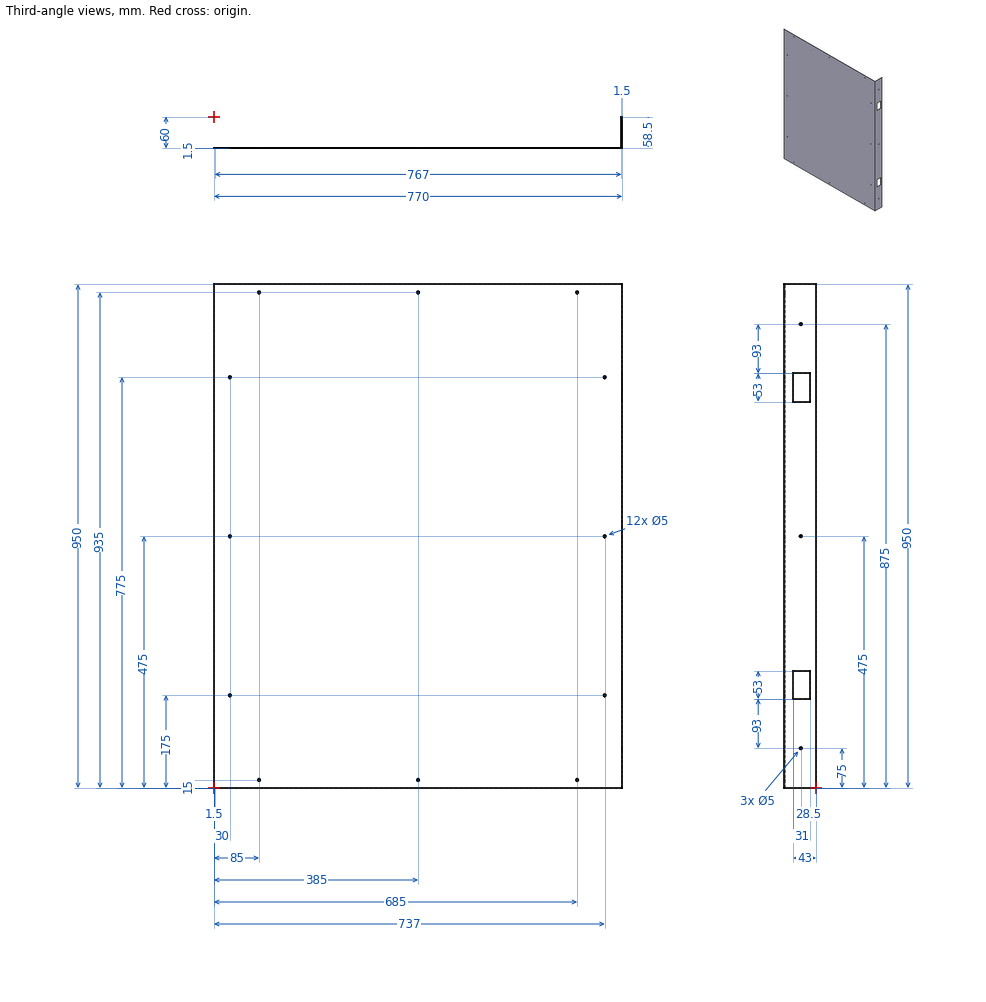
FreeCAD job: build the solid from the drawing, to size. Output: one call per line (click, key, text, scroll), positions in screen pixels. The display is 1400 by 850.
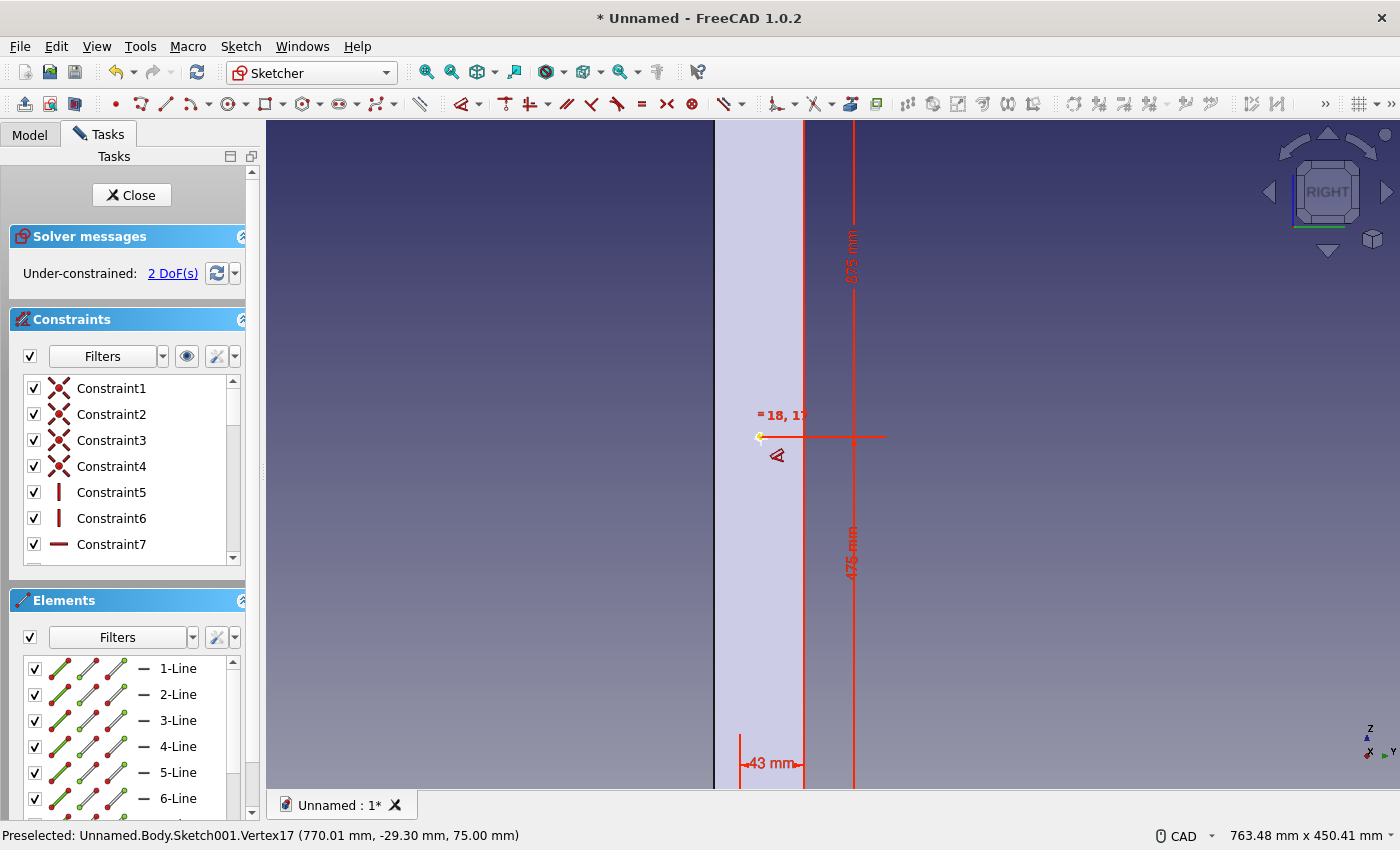
click(760, 437)
click(782, 403)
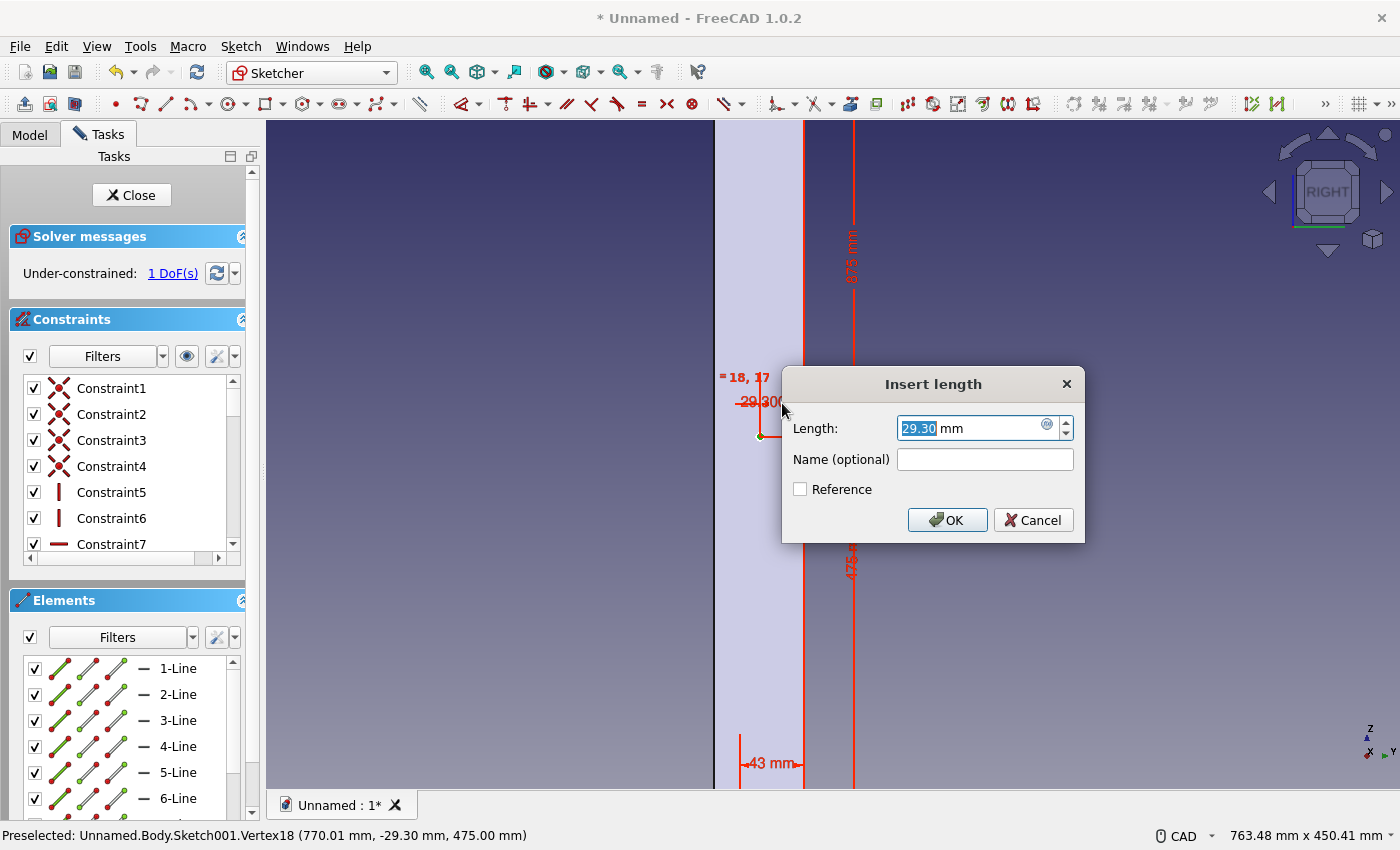
text(28.5)
key(Return)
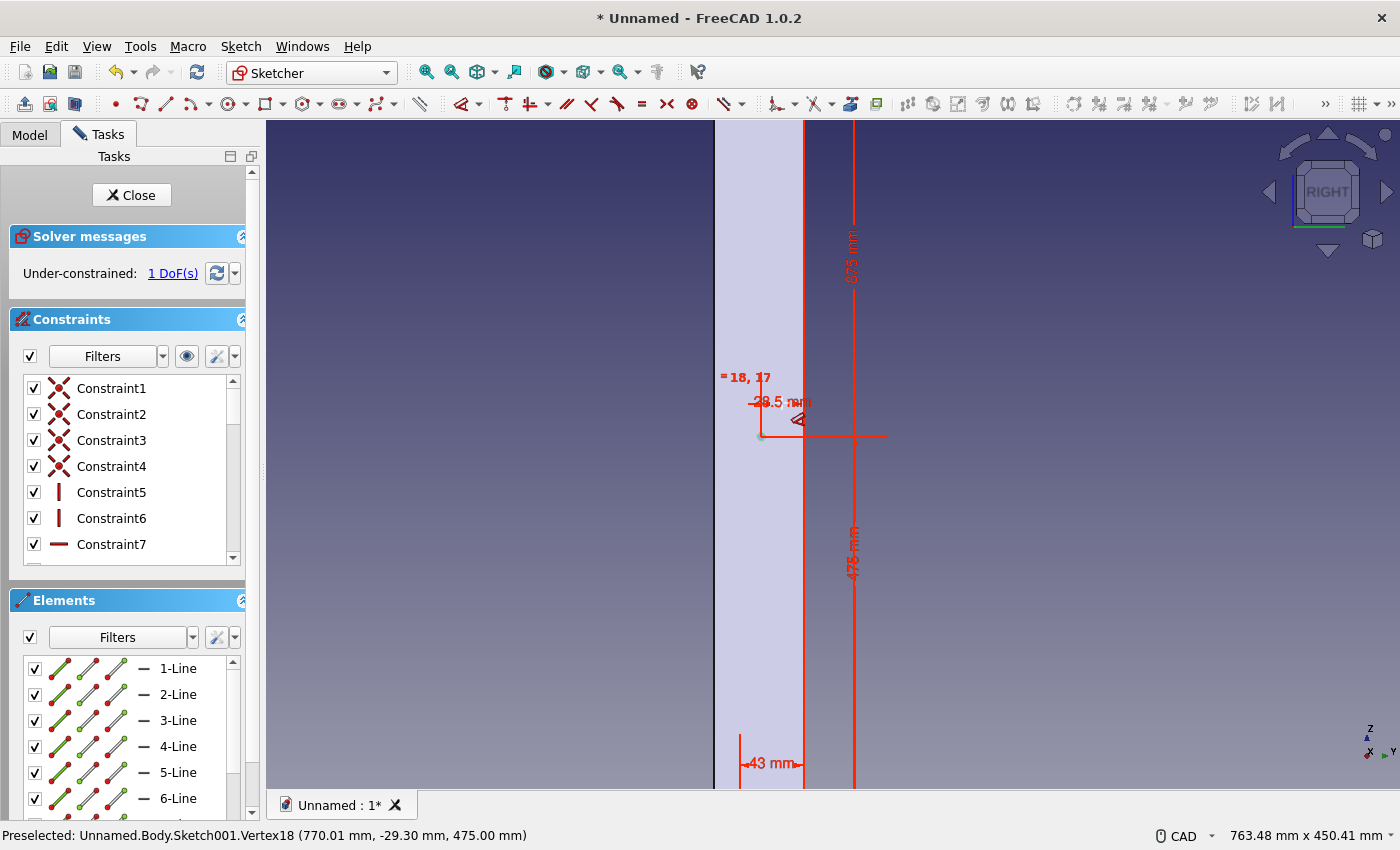
scroll(761, 439, down, 6)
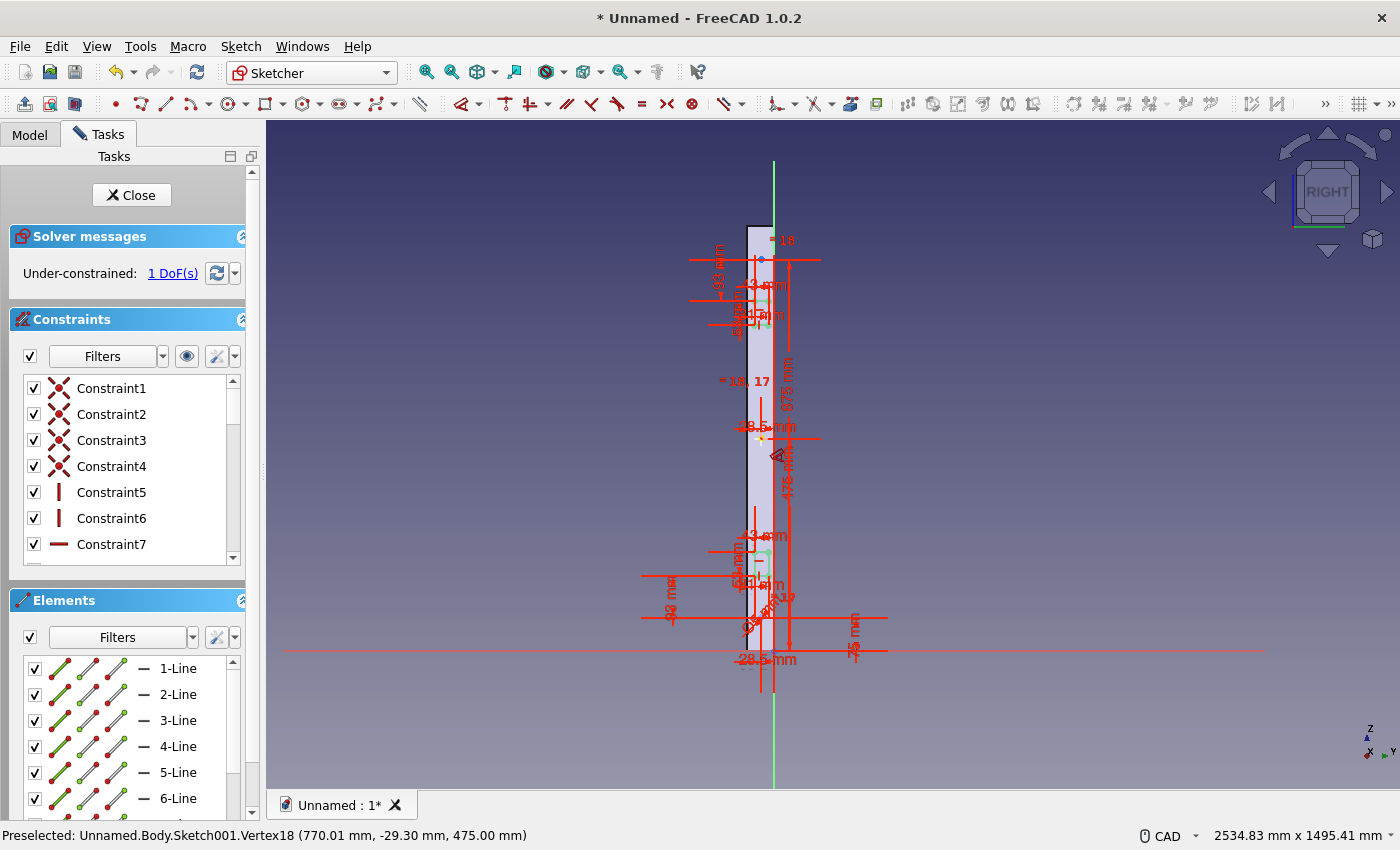
scroll(761, 260, up, 6)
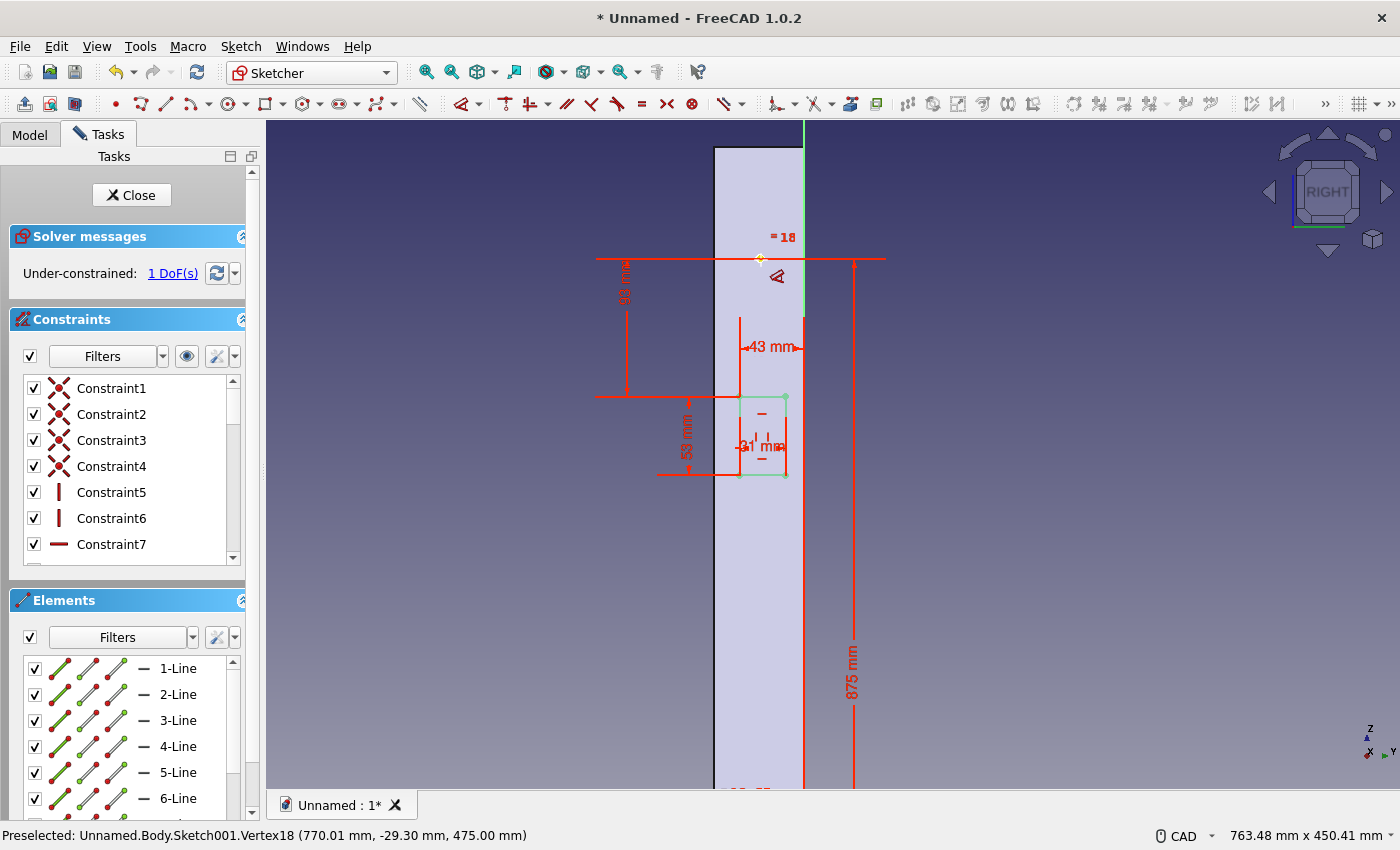
click(760, 259)
click(782, 225)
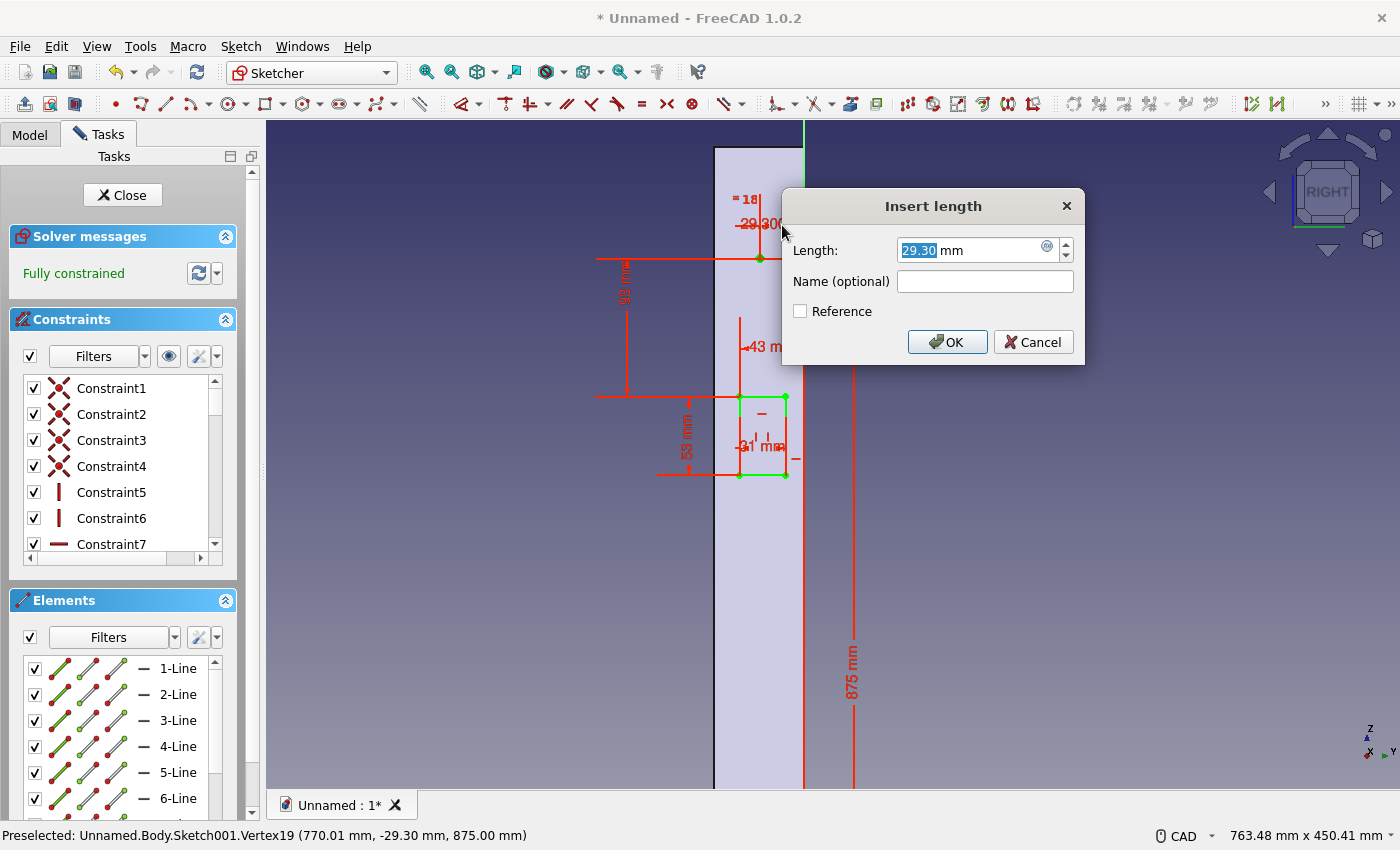
text(28.5)
key(Return)
key(Escape)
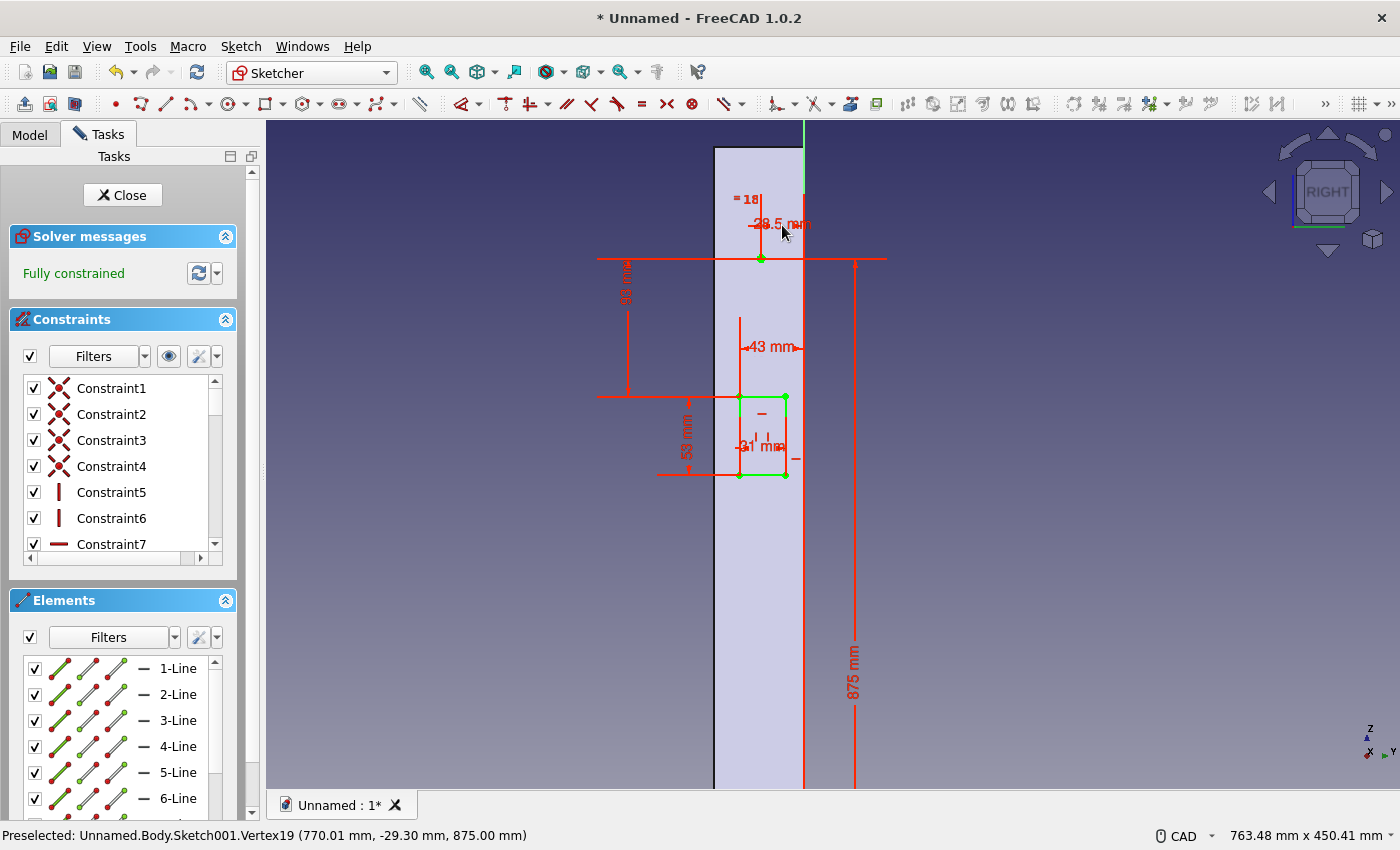
click(123, 195)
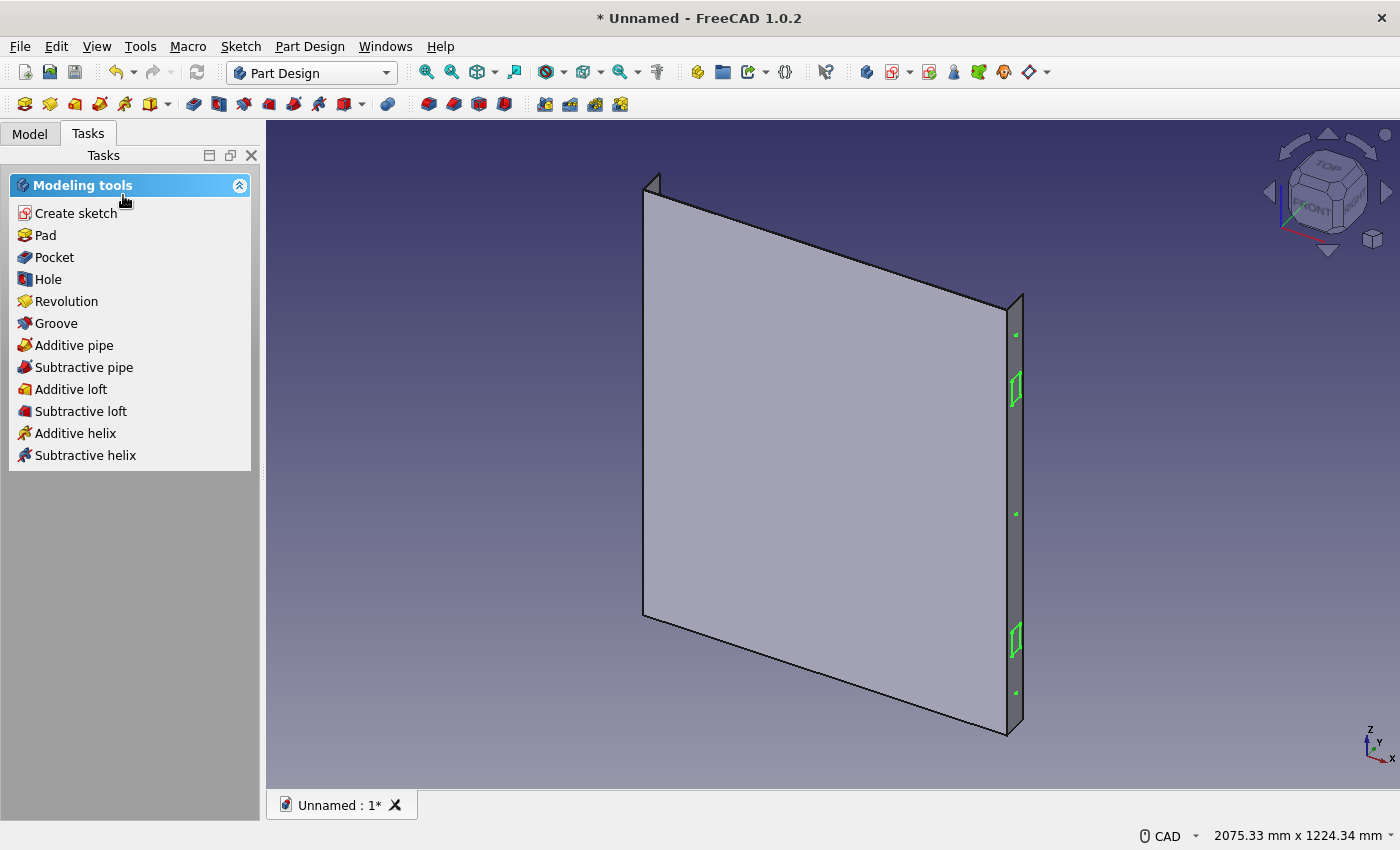
click(194, 104)